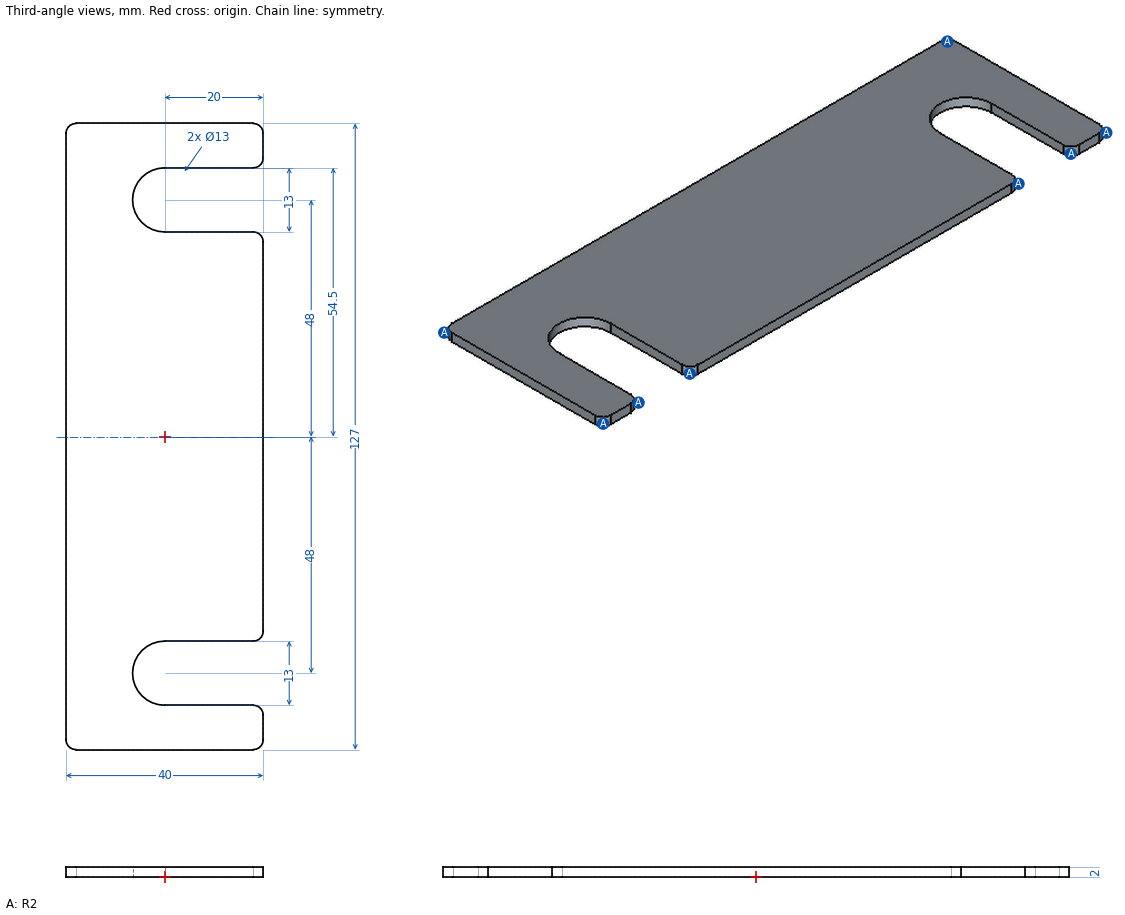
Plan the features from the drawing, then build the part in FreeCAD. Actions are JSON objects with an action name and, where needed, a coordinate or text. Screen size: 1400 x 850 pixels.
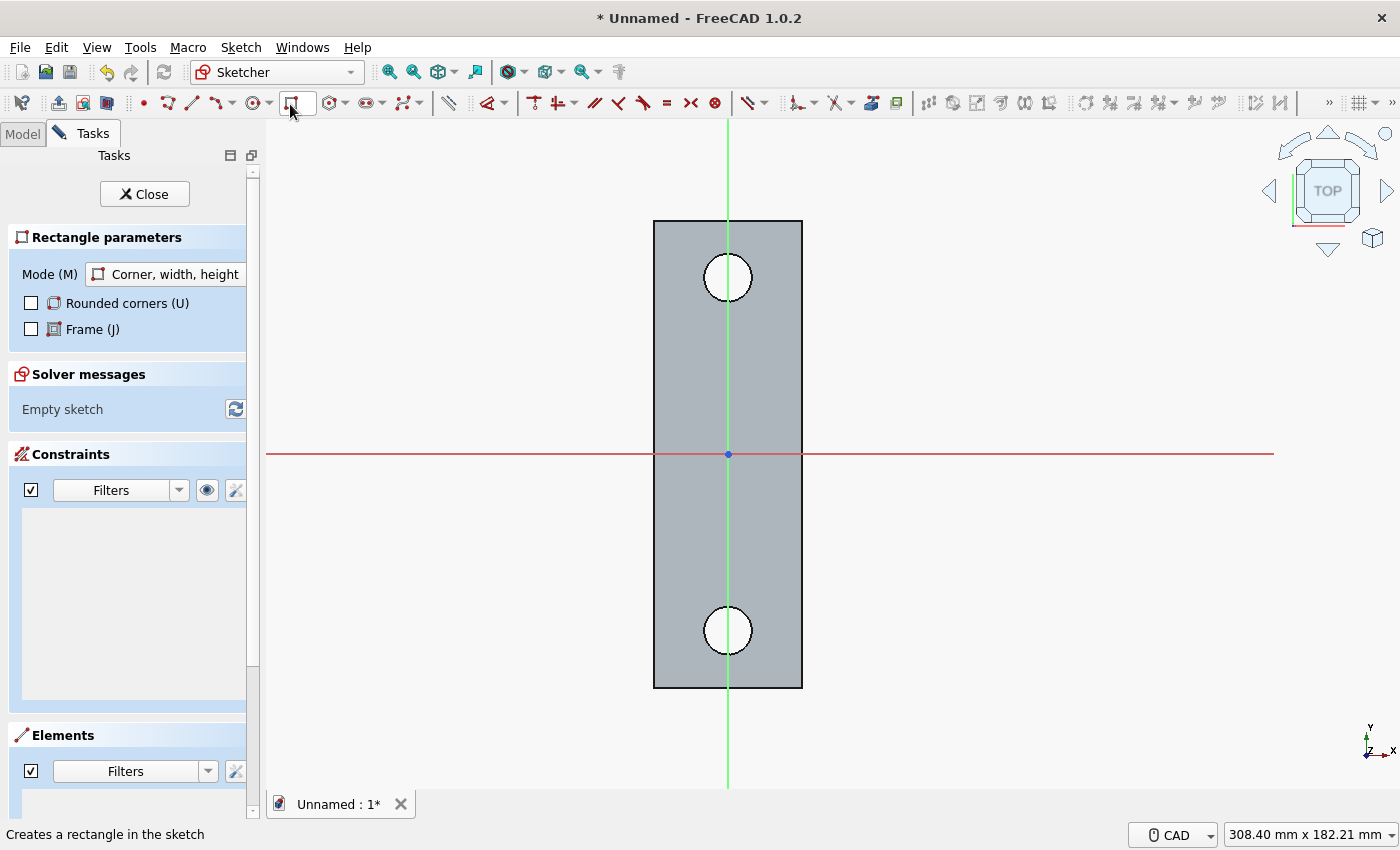
{"action": "left_click", "coordinate": [728, 254]}
{"action": "left_click", "coordinate": [802, 302]}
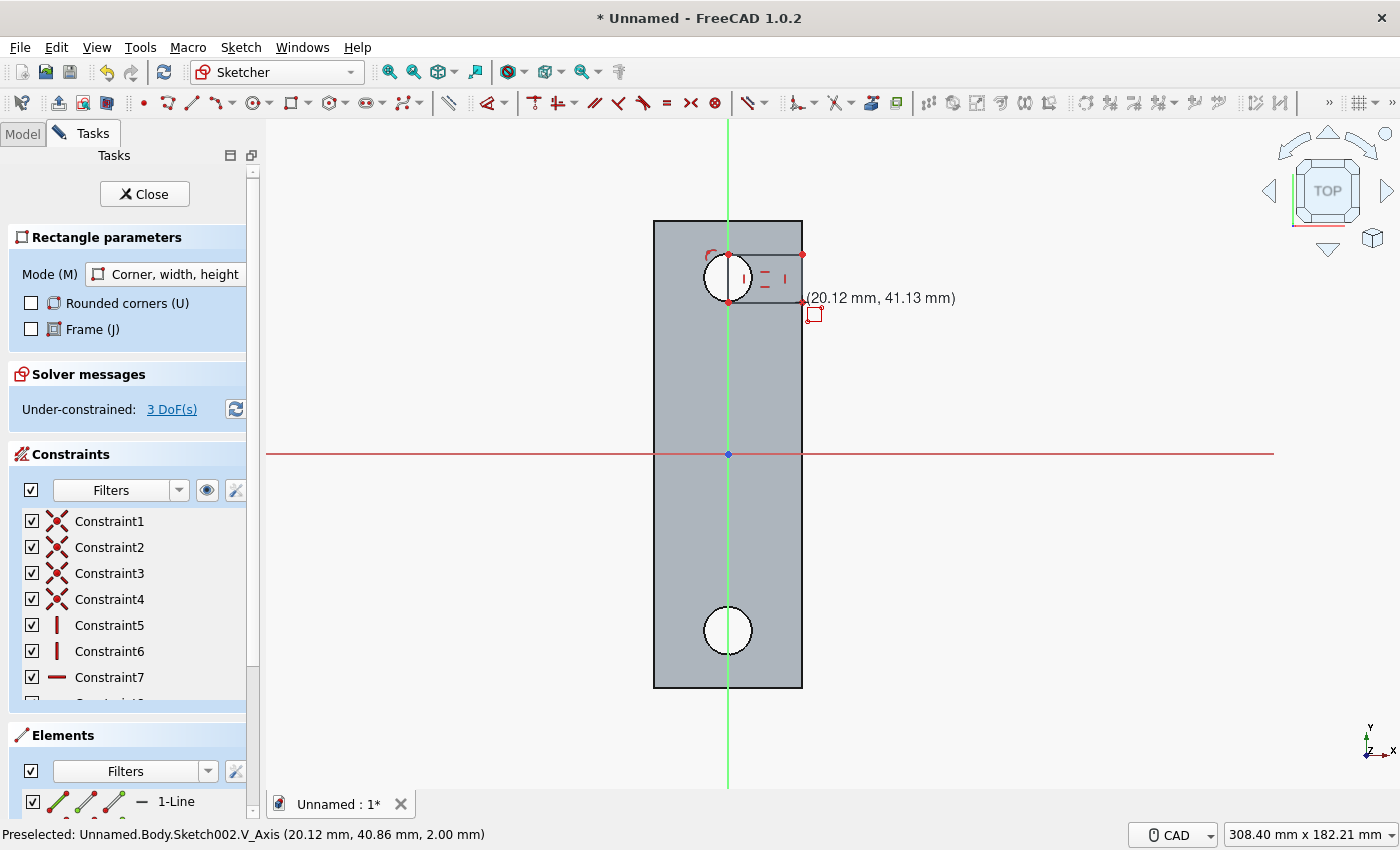
{"action": "left_click", "coordinate": [728, 607]}
{"action": "left_click", "coordinate": [802, 655]}
{"action": "key", "text": "Escape"}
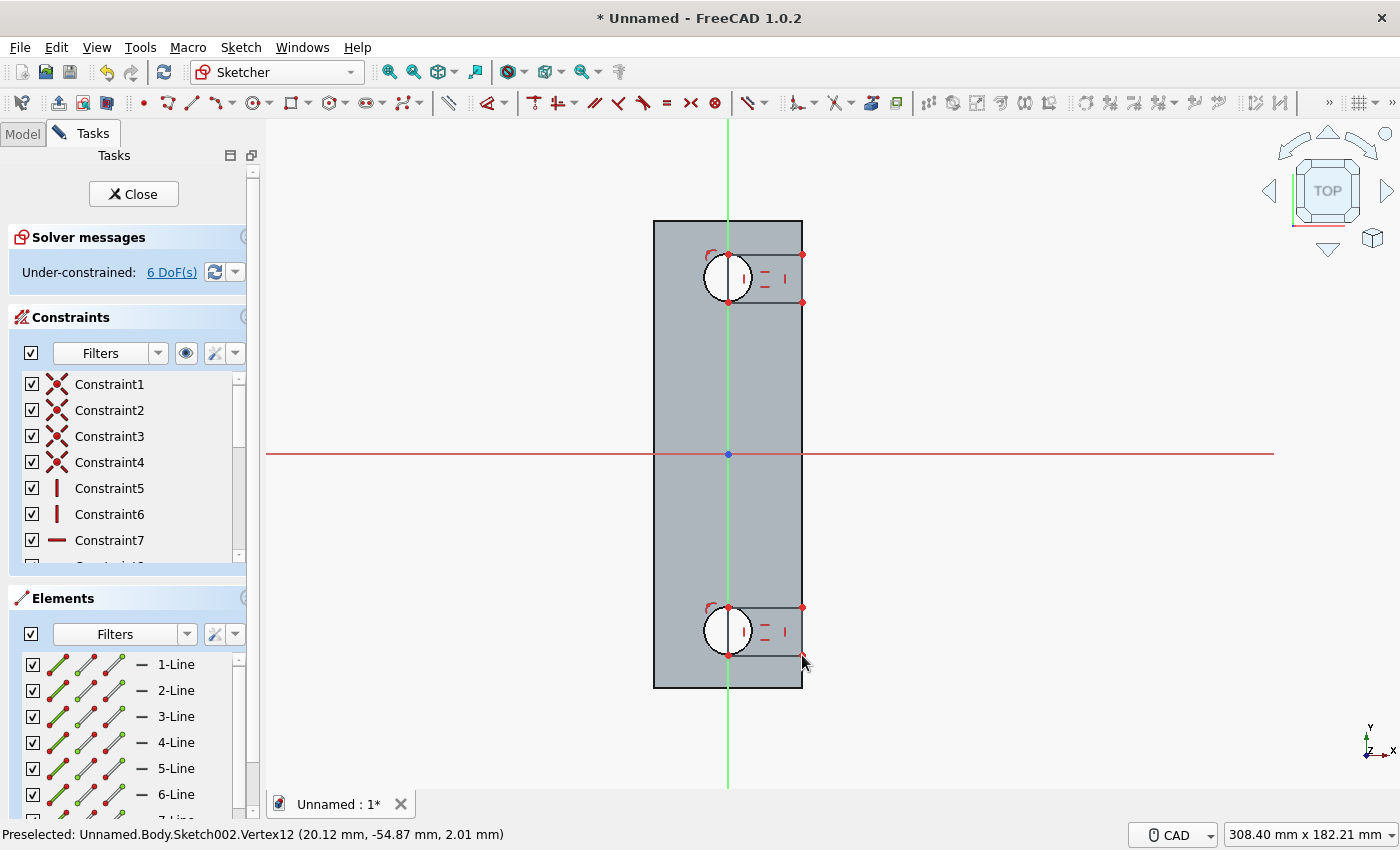
{"action": "left_click", "coordinate": [802, 255]}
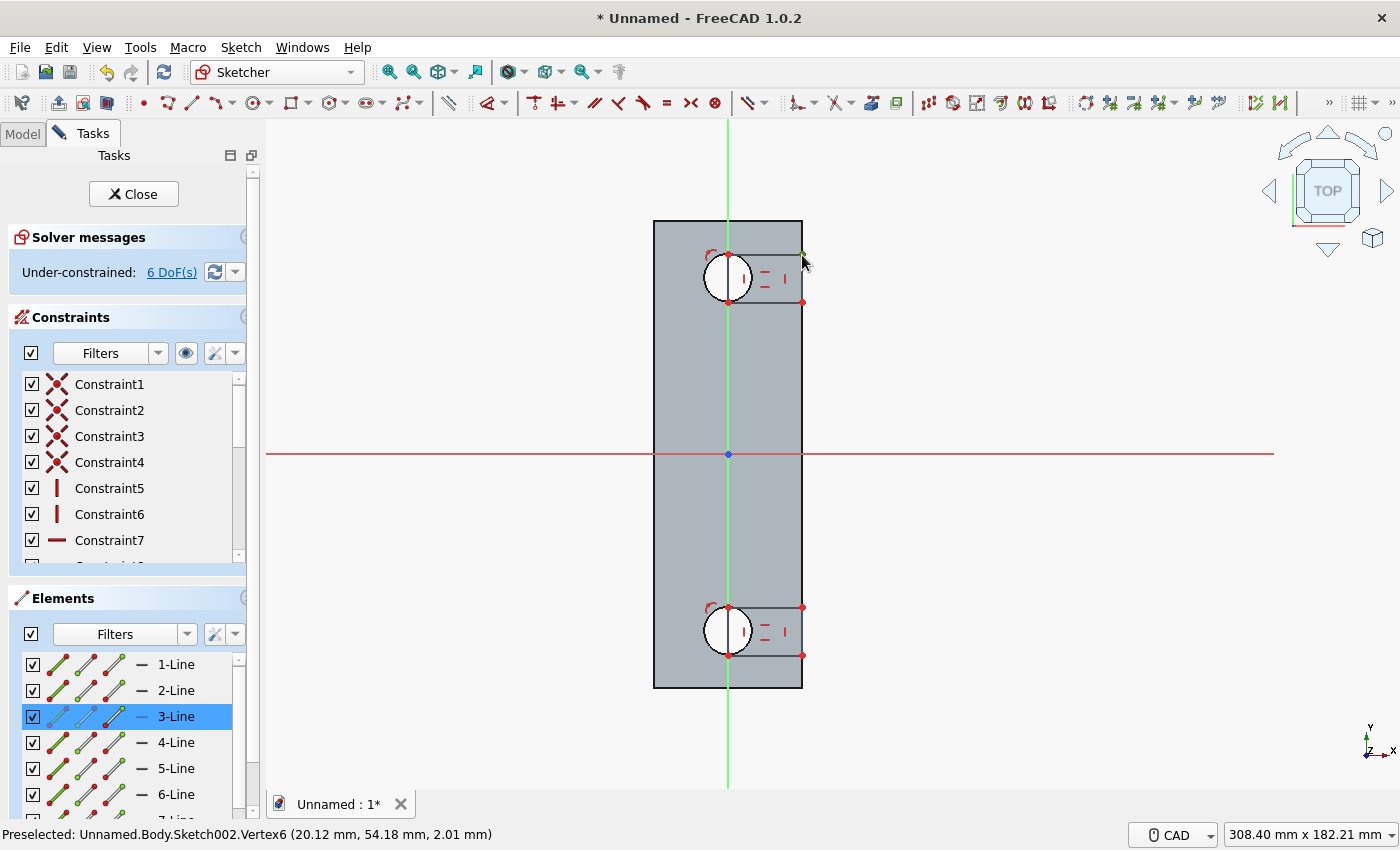
{"action": "left_click", "coordinate": [802, 656]}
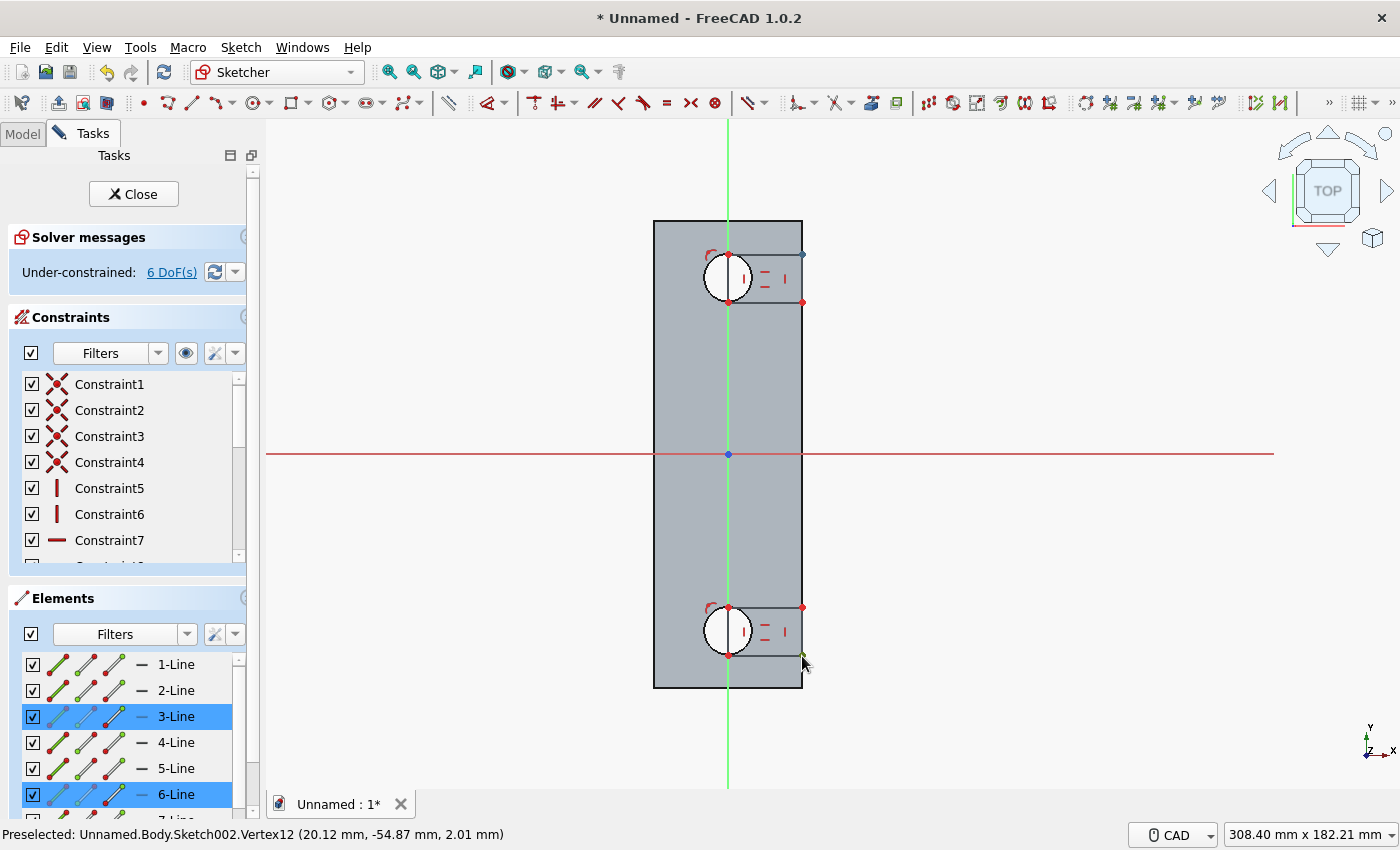
{"action": "left_click", "coordinate": [361, 454]}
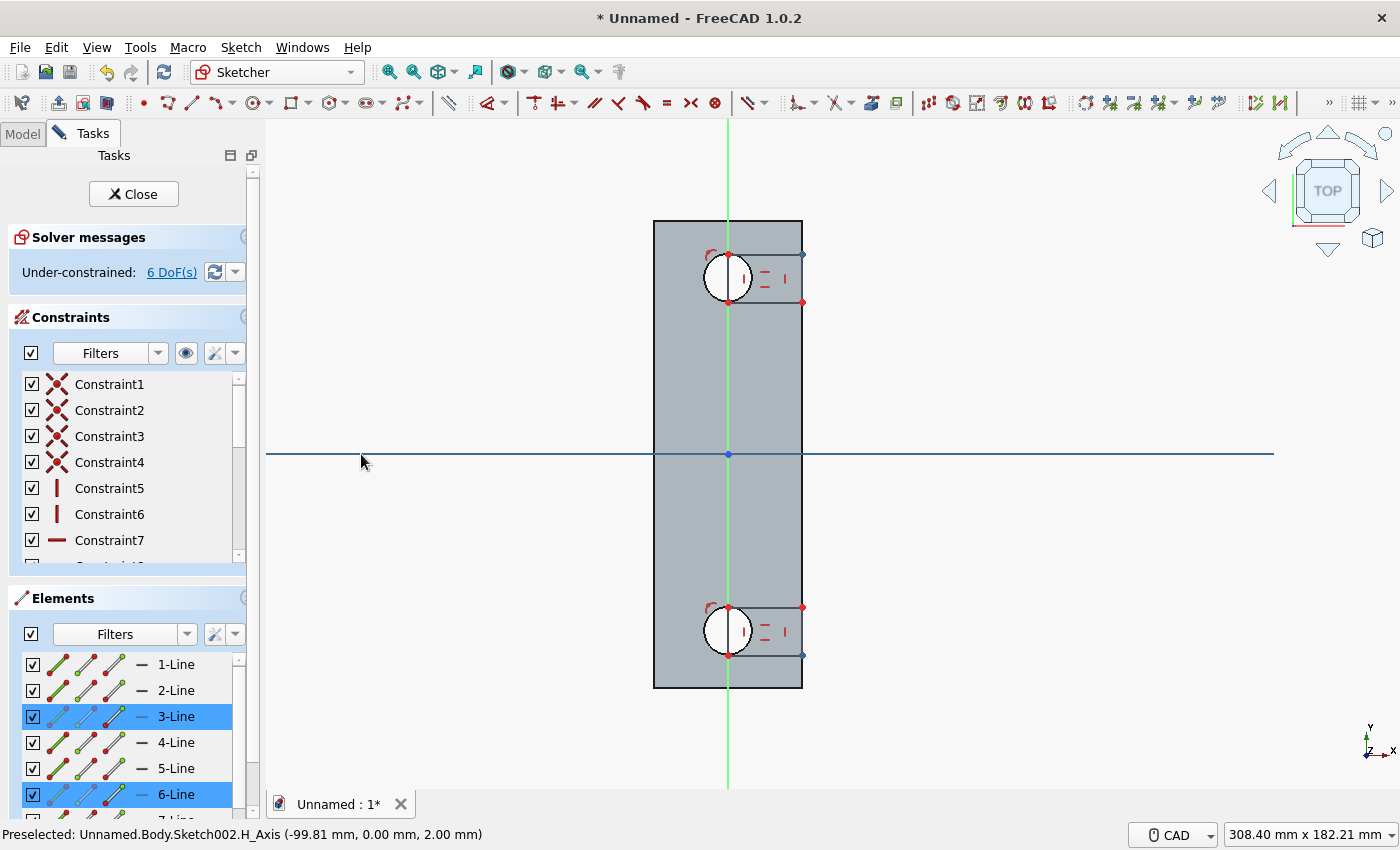
{"action": "left_click", "coordinate": [692, 104]}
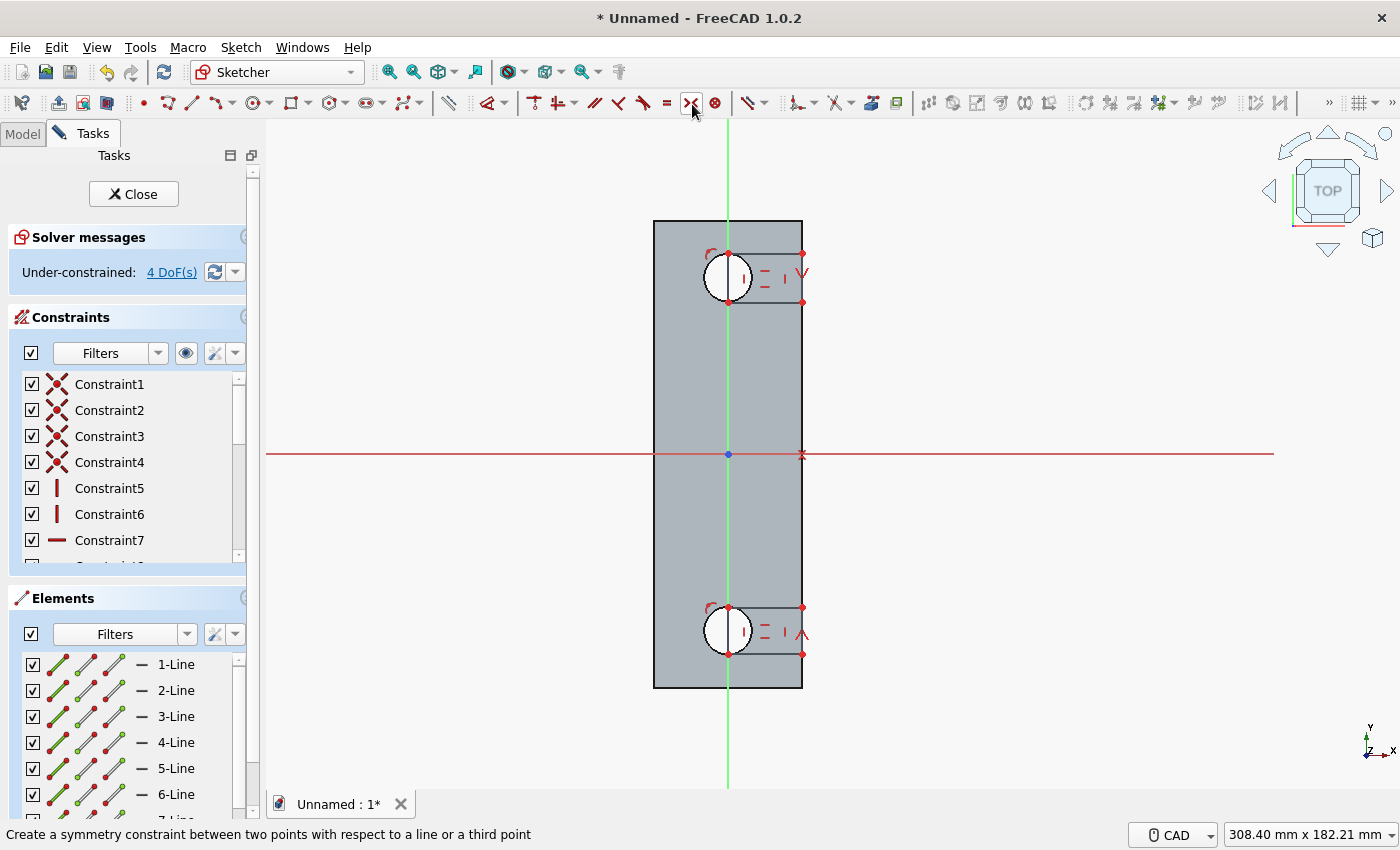
{"action": "left_click", "coordinate": [488, 104]}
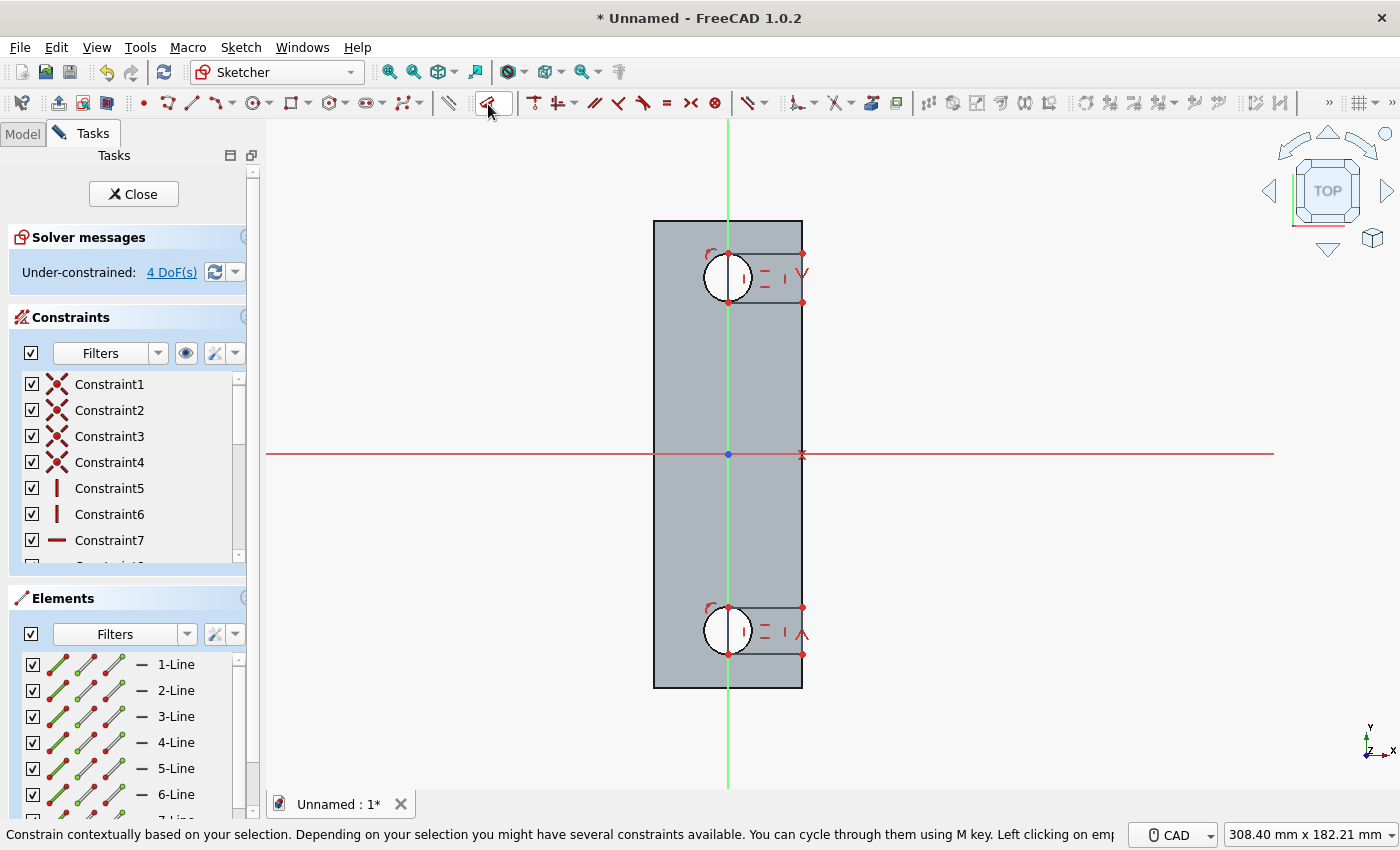
{"action": "left_click", "coordinate": [728, 269]}
{"action": "left_click", "coordinate": [694, 278]}